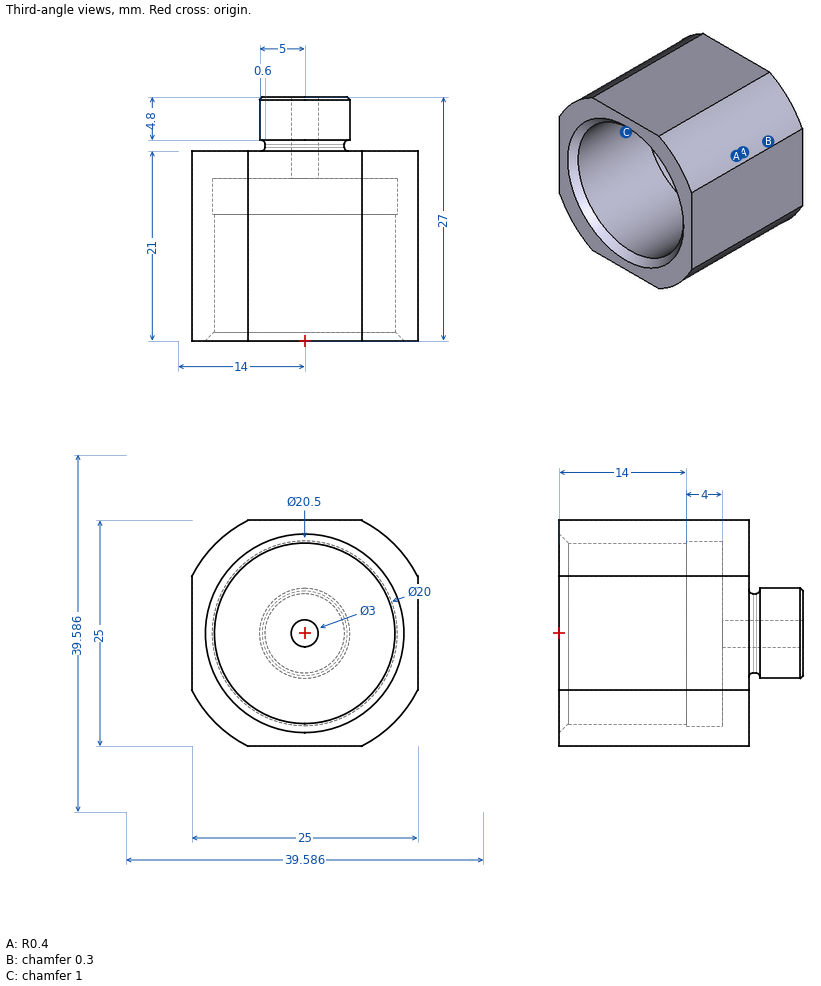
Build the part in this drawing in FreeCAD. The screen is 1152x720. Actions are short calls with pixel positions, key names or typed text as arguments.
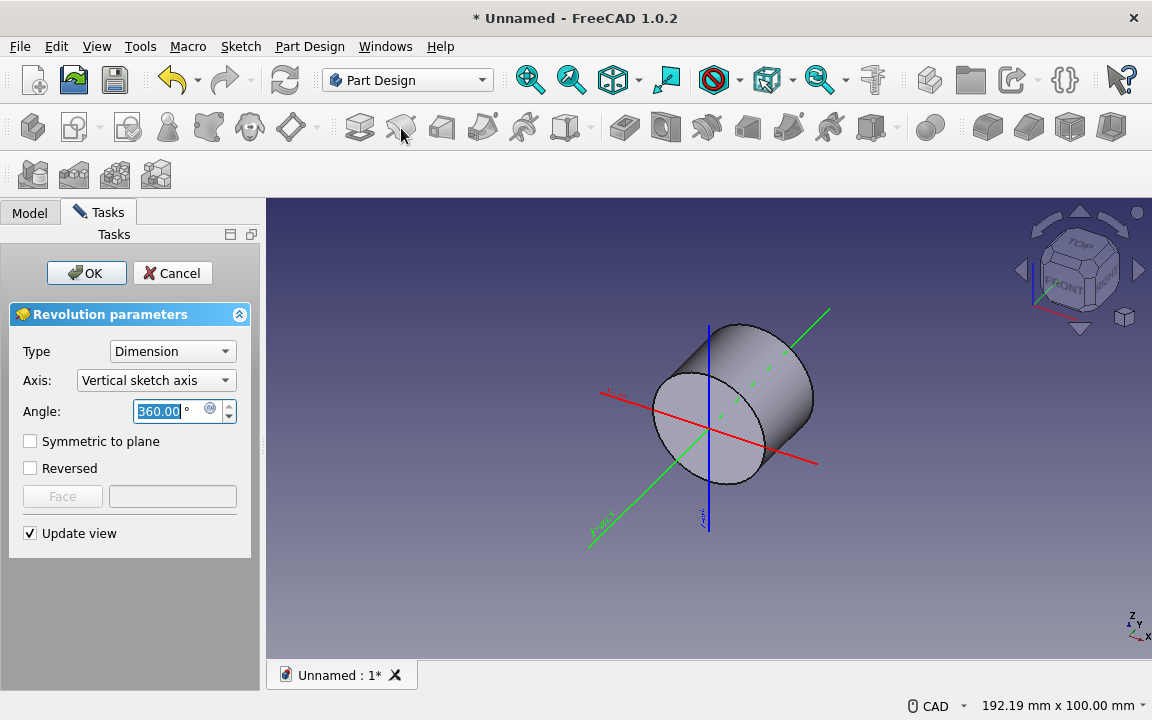
click(87, 273)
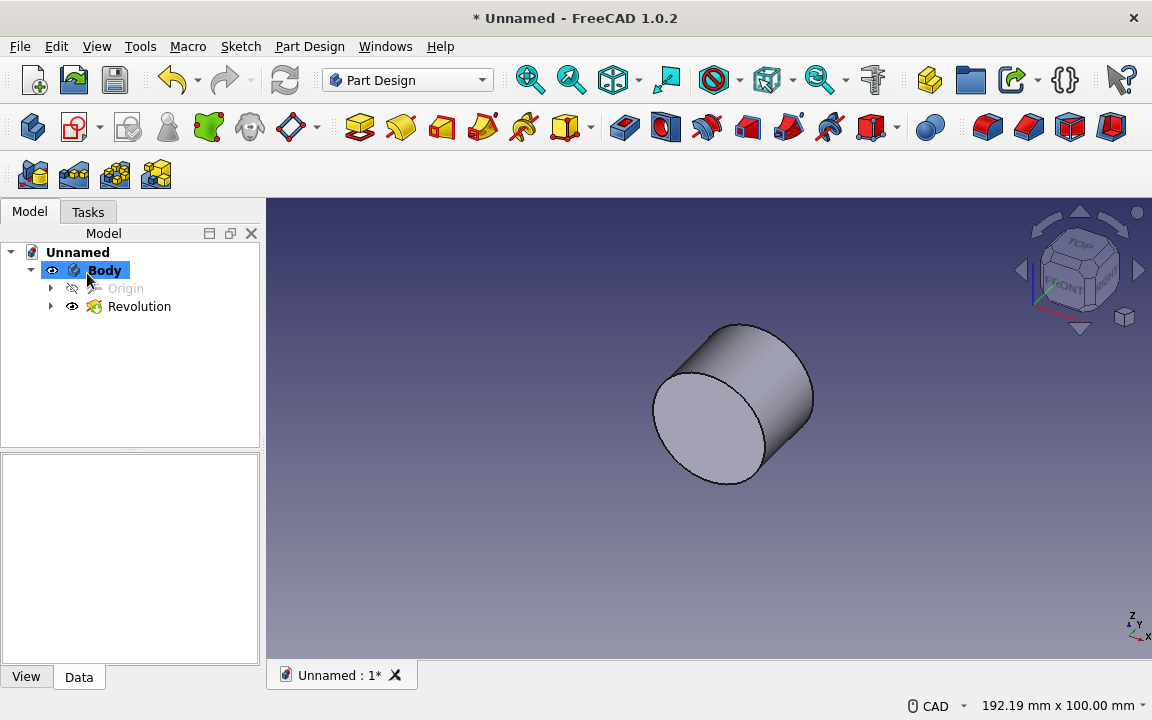
click(531, 80)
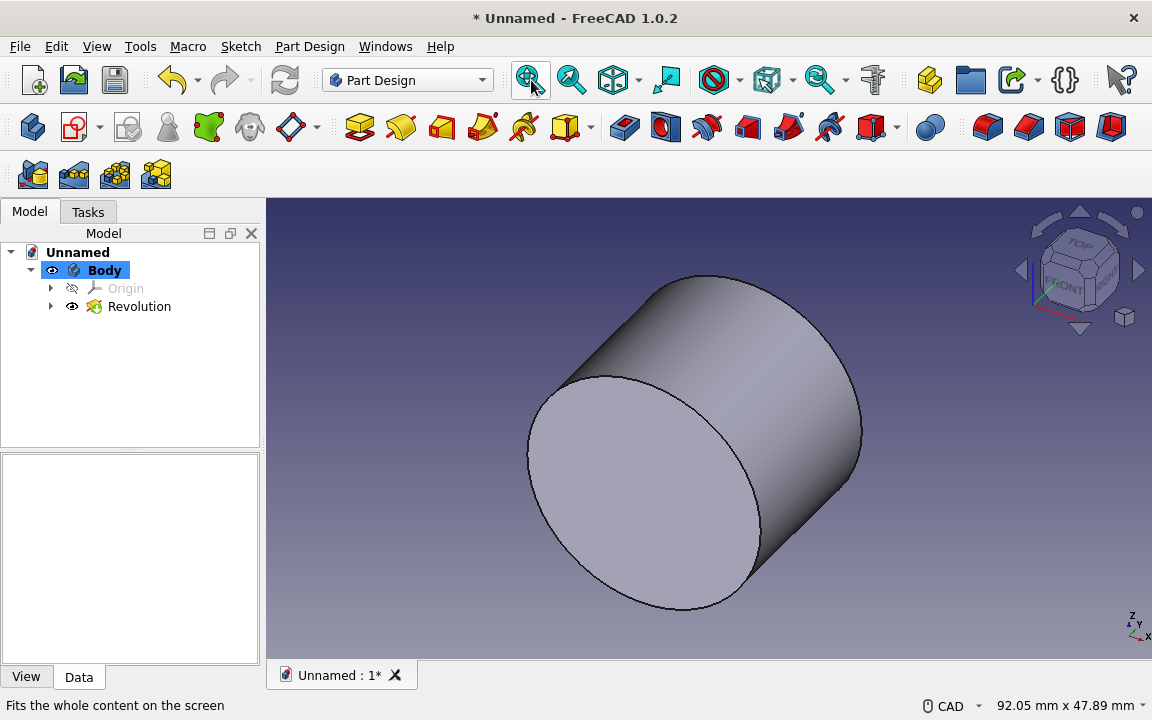
key(0)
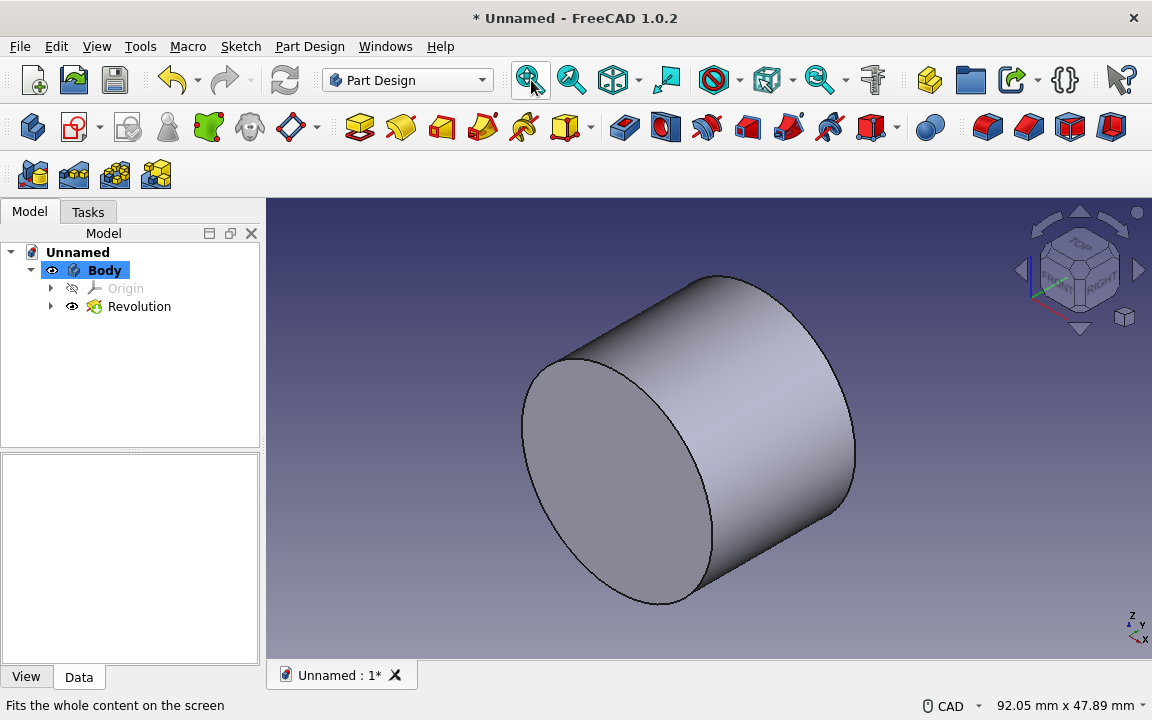
key(2)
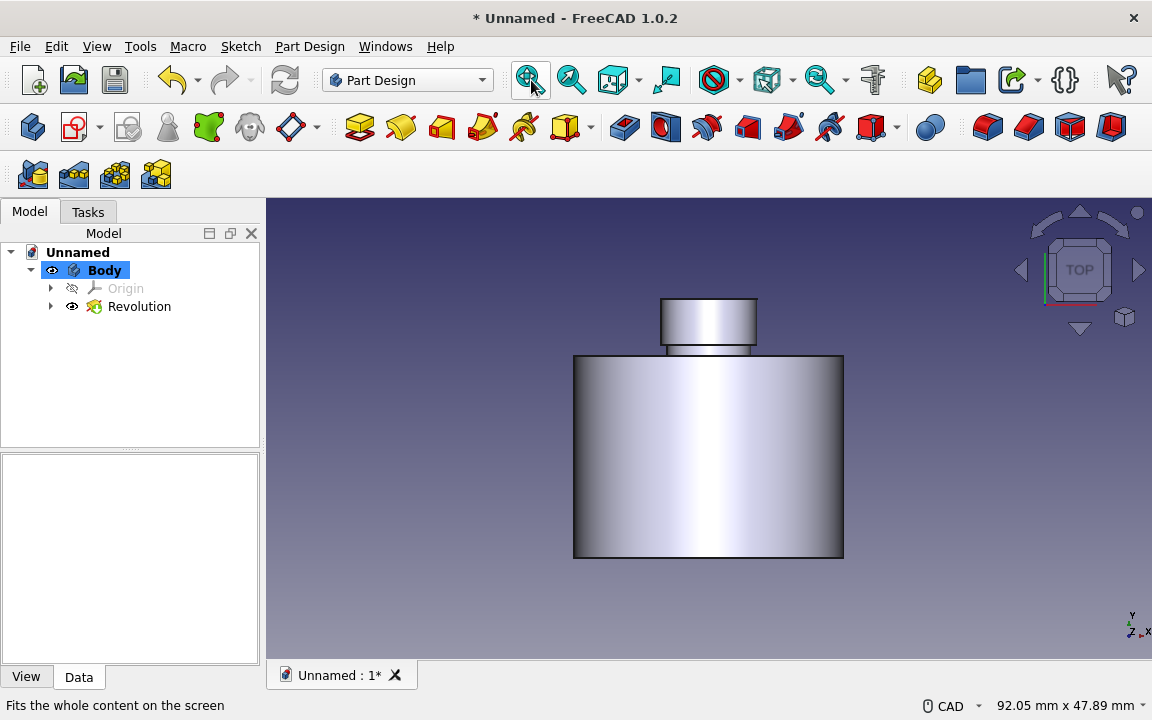
key(1)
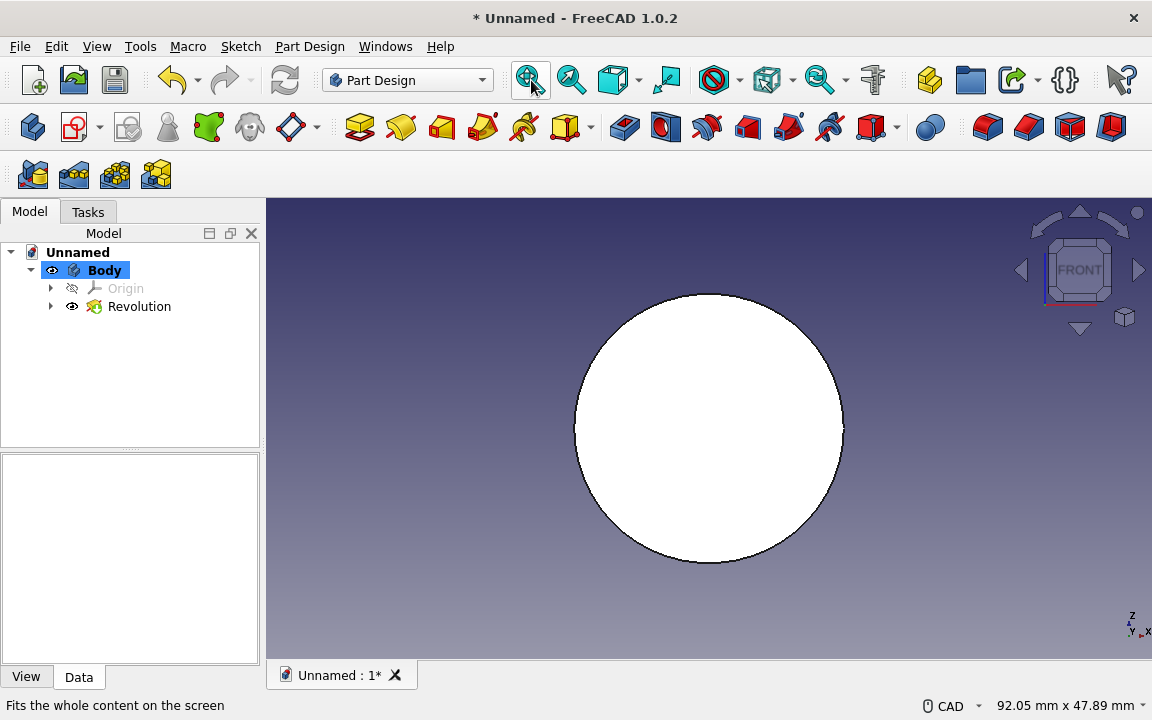
key(3)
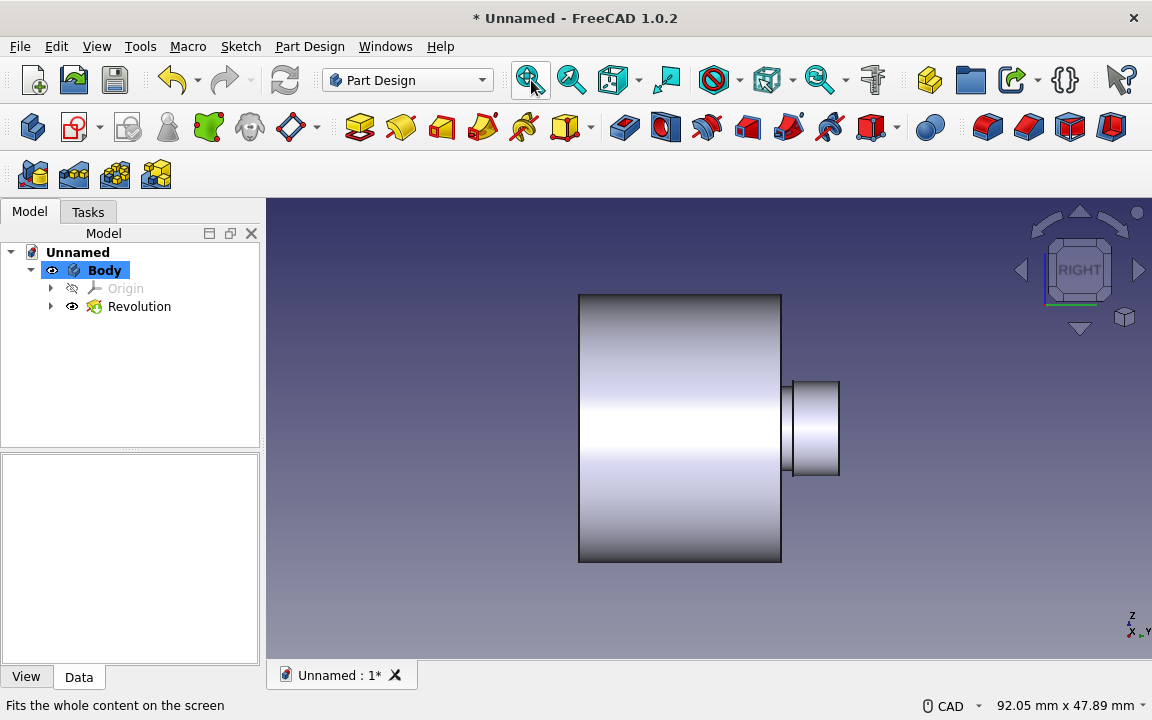
key(5)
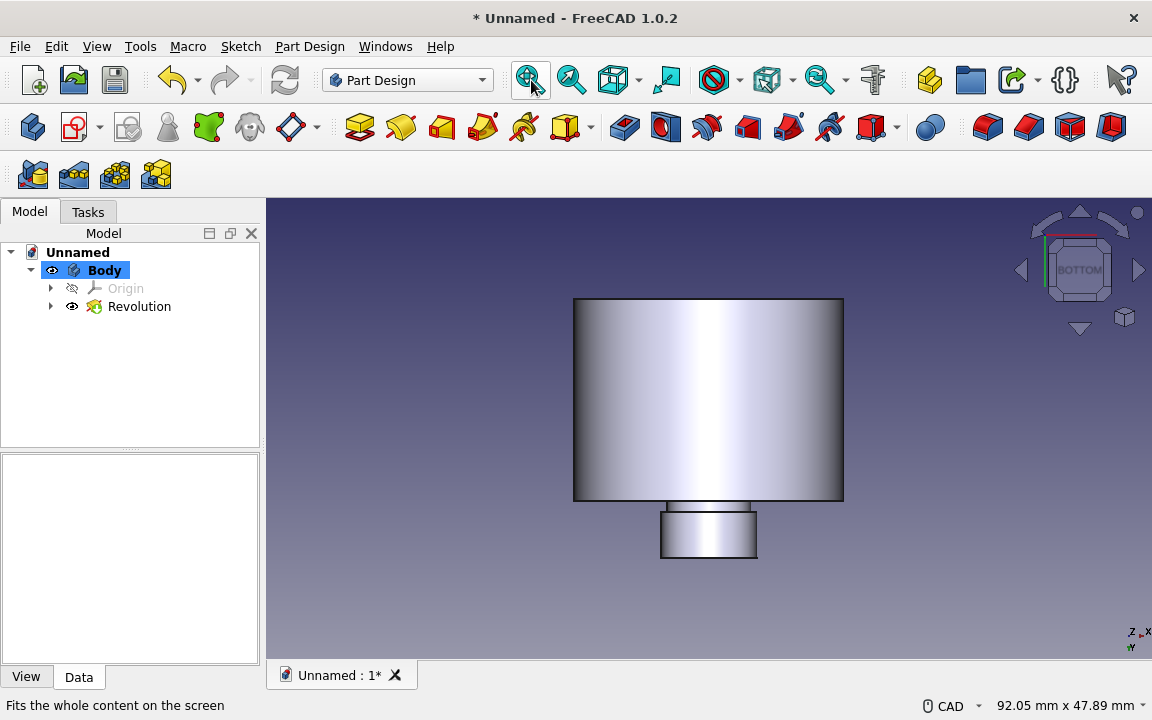
key(4)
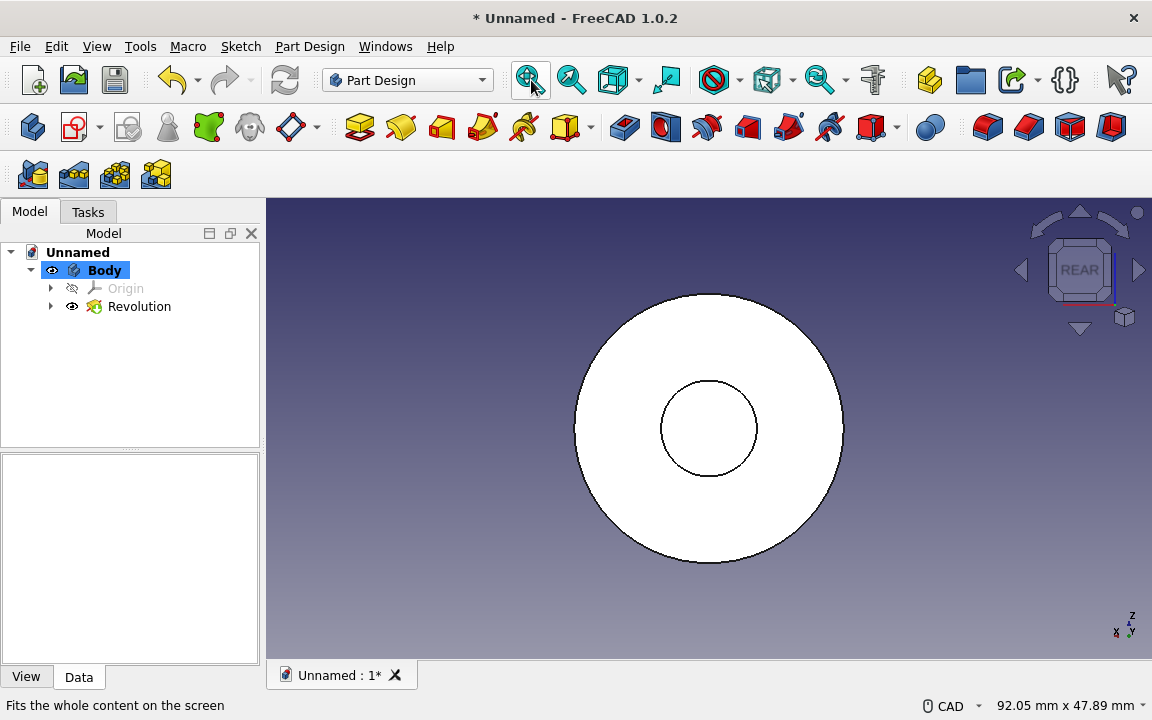
key(6)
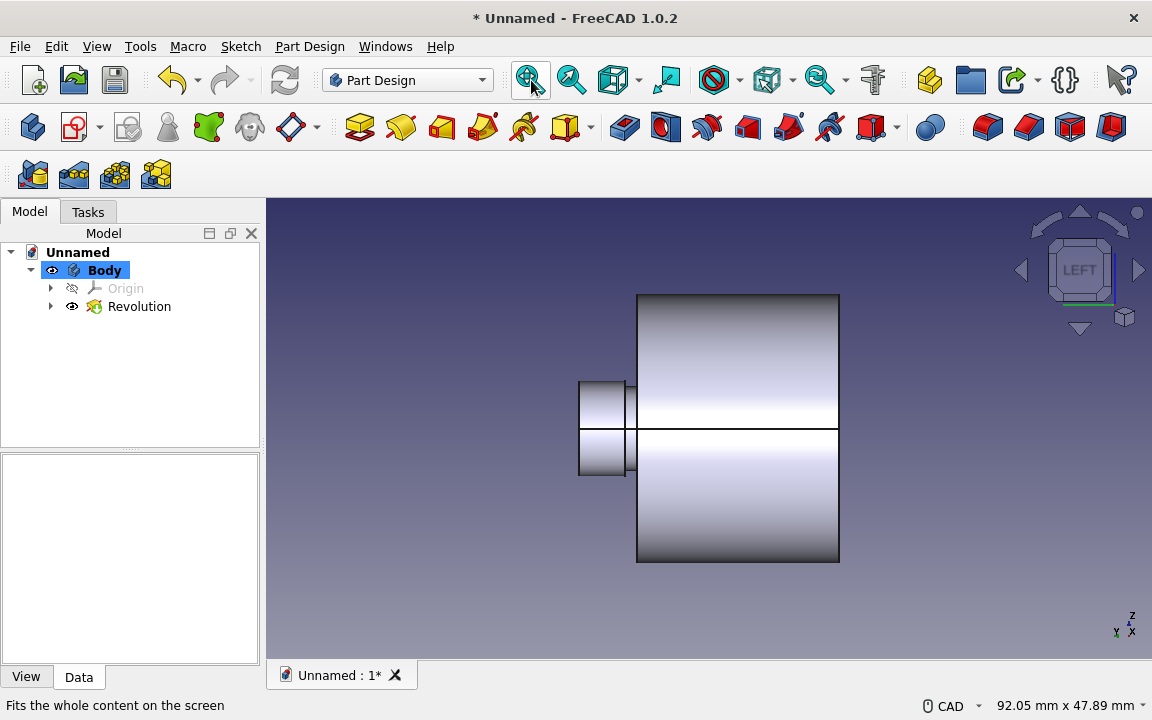
key(v)
key(3)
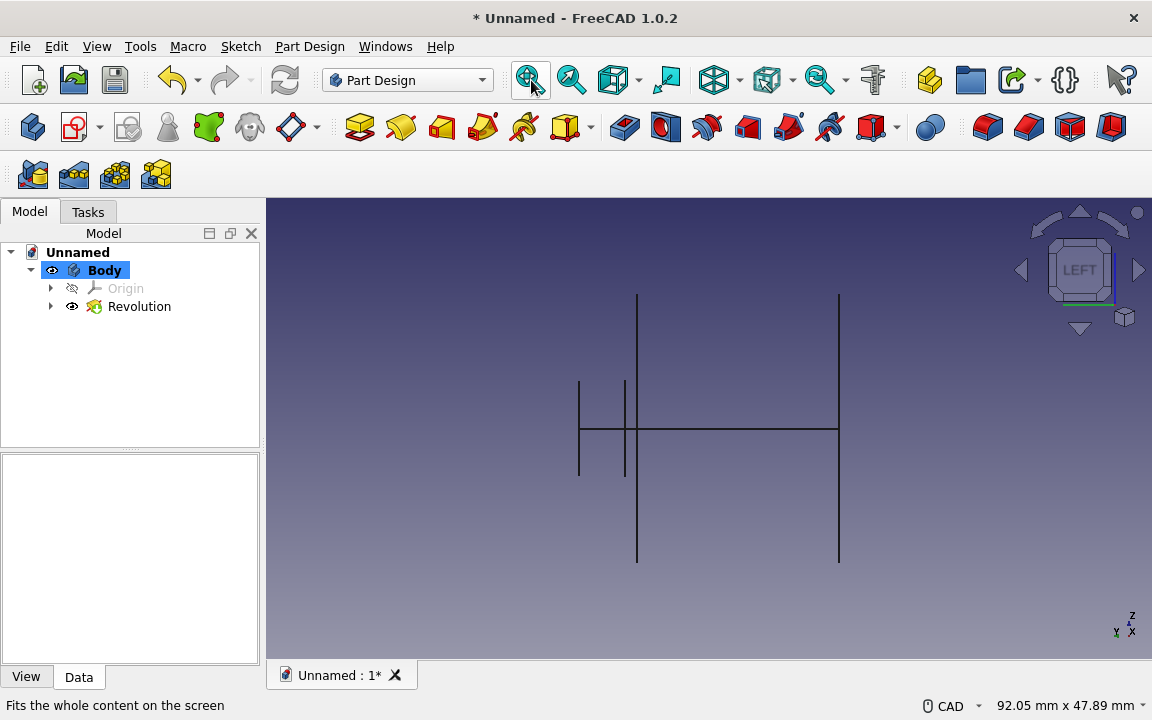
key(0)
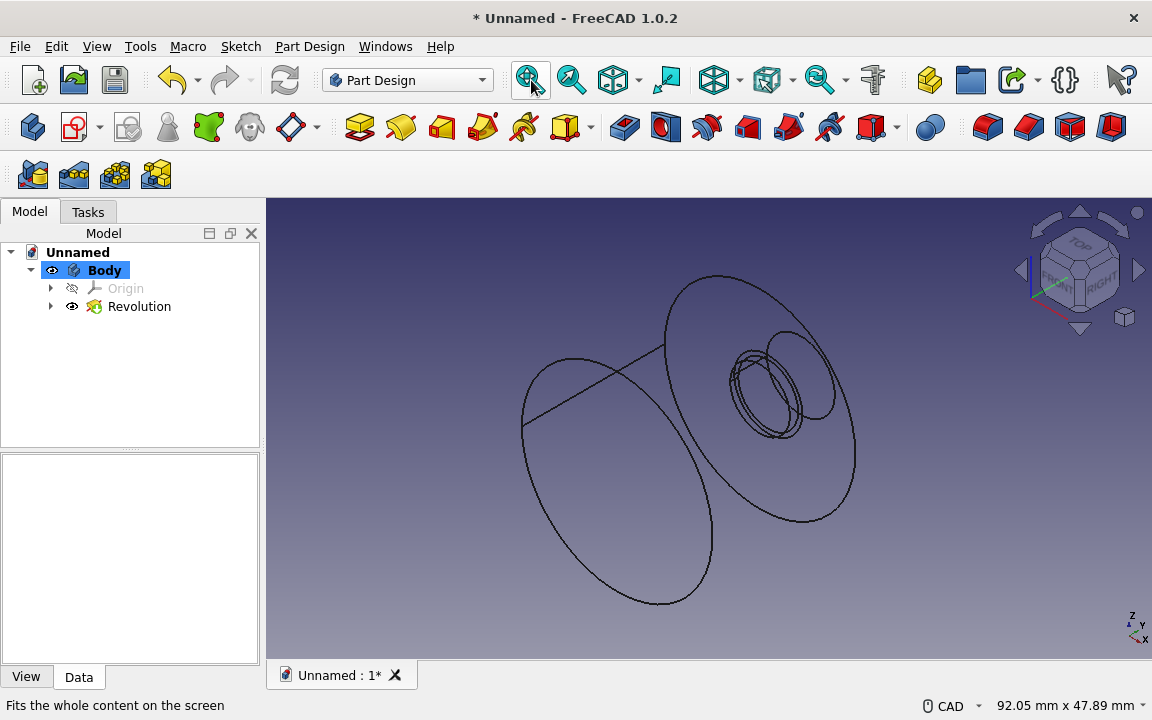
click(759, 421)